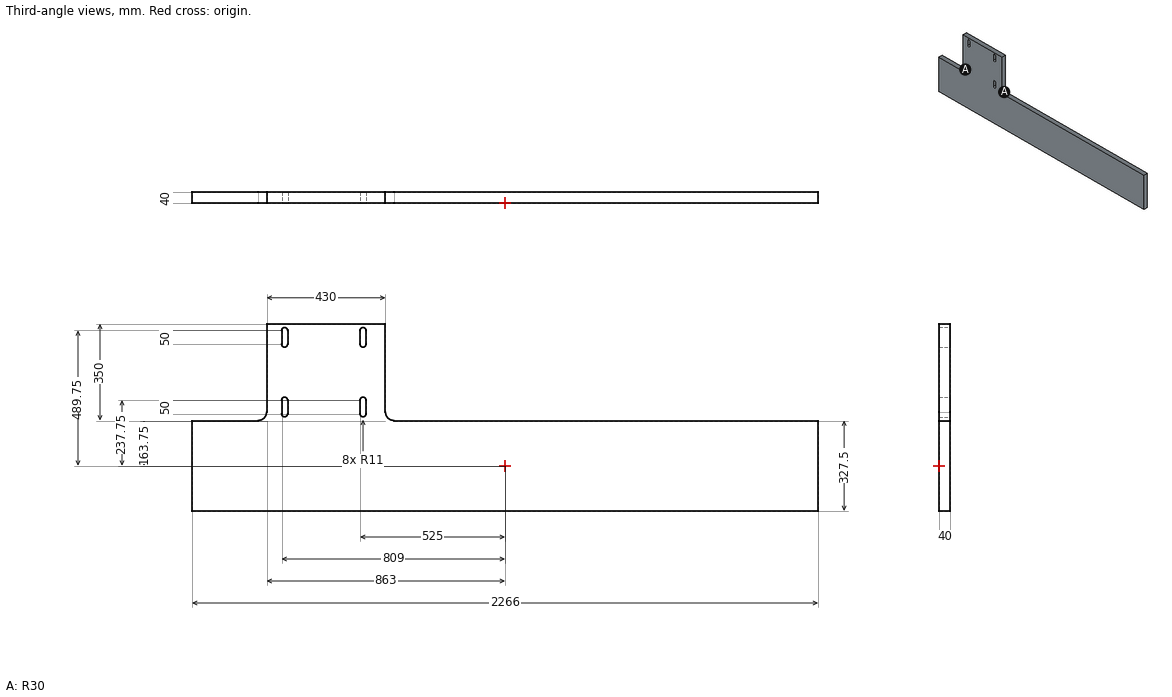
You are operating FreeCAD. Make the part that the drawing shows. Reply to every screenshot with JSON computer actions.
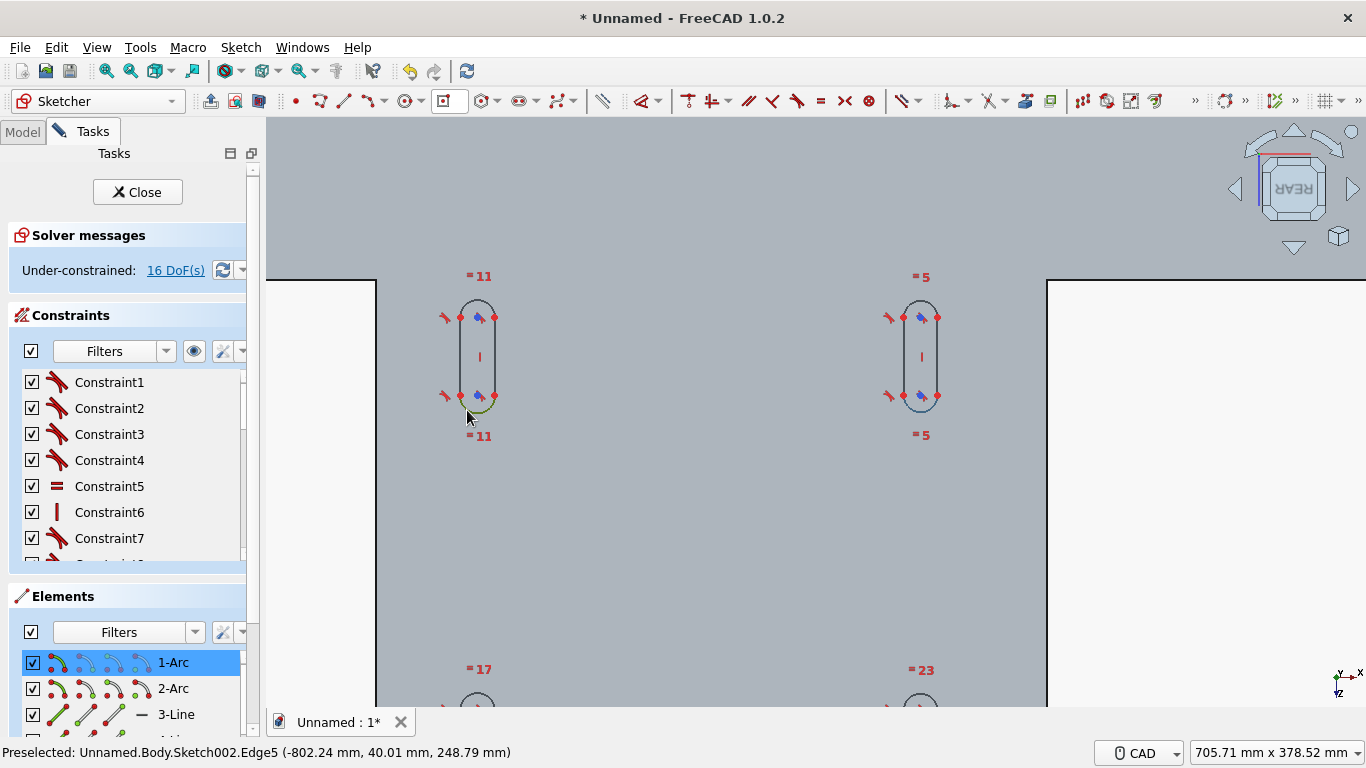
{"action": "scroll", "coordinate": [467, 410], "scroll_direction": "down", "scroll_amount": 4}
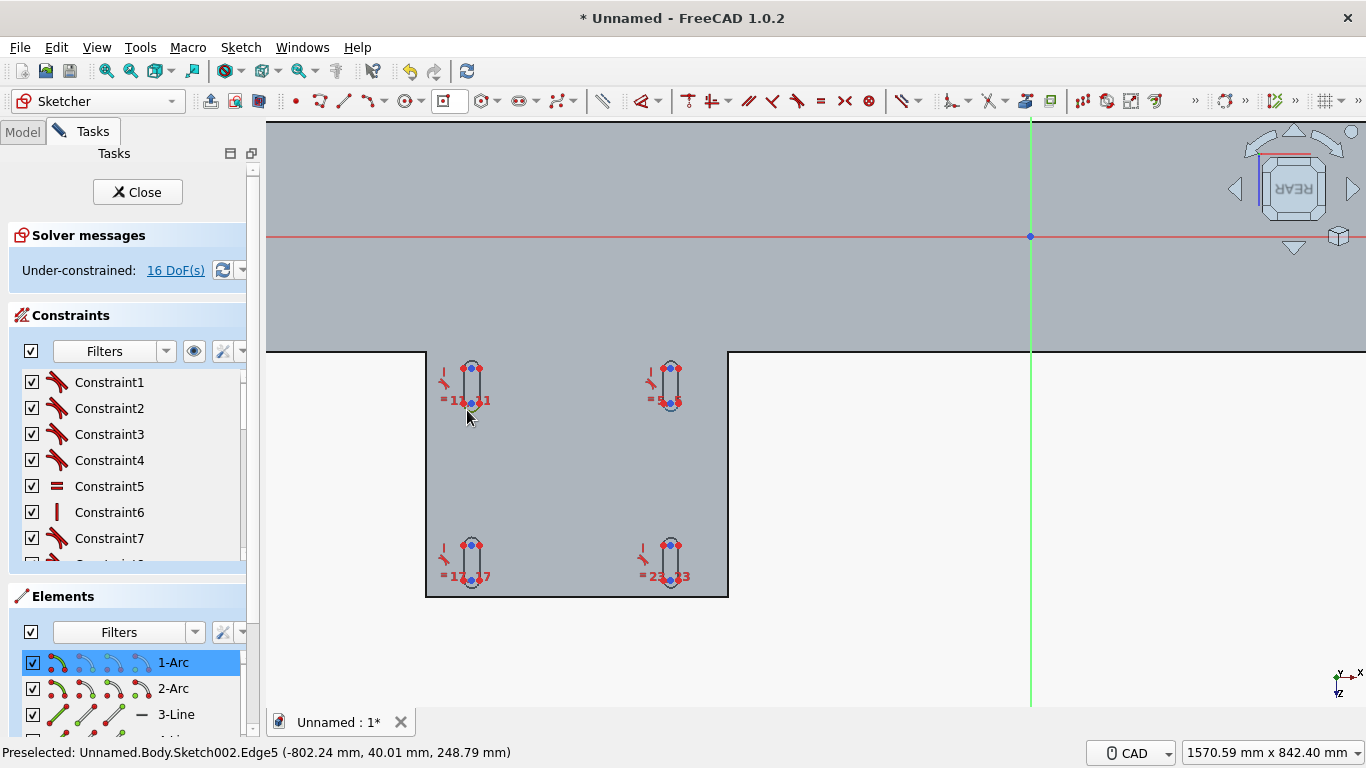
{"action": "scroll", "coordinate": [467, 587], "scroll_direction": "up", "scroll_amount": 4}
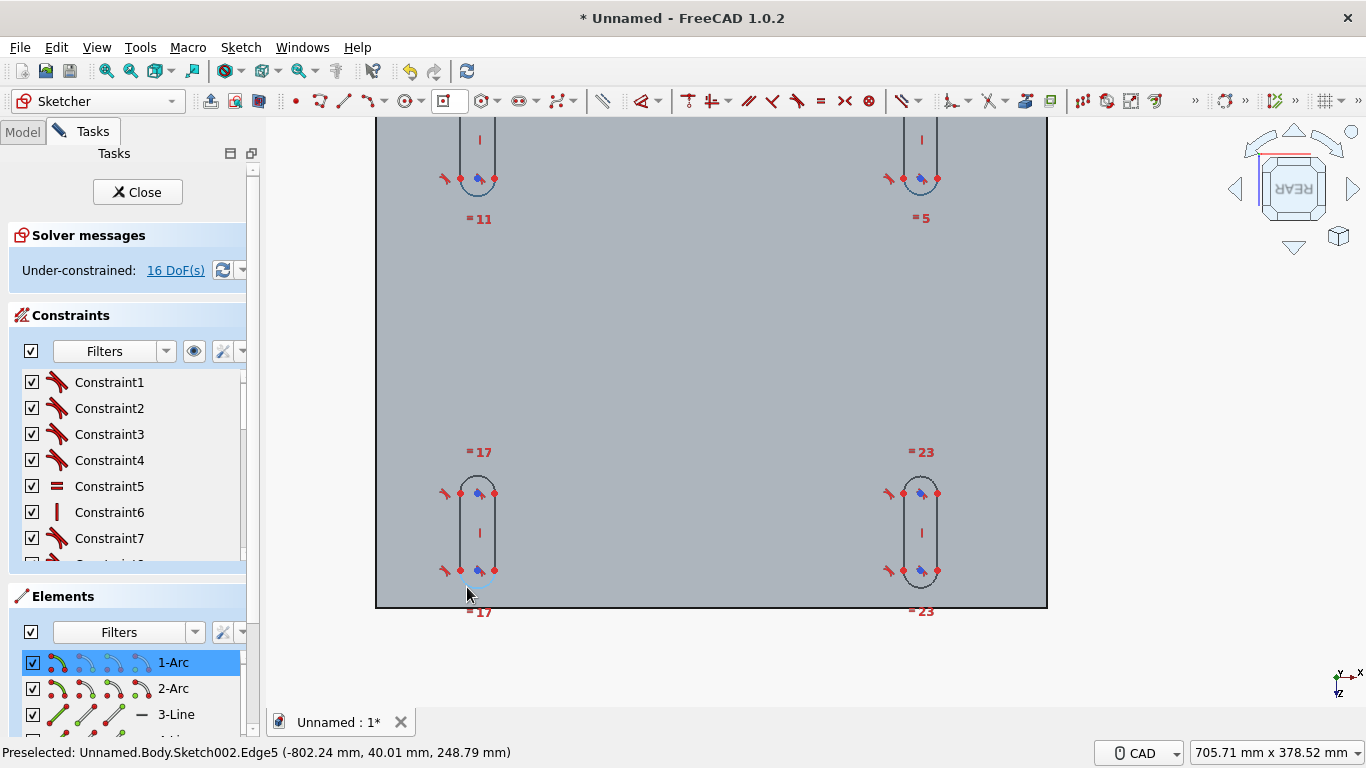
{"action": "left_click", "coordinate": [467, 585]}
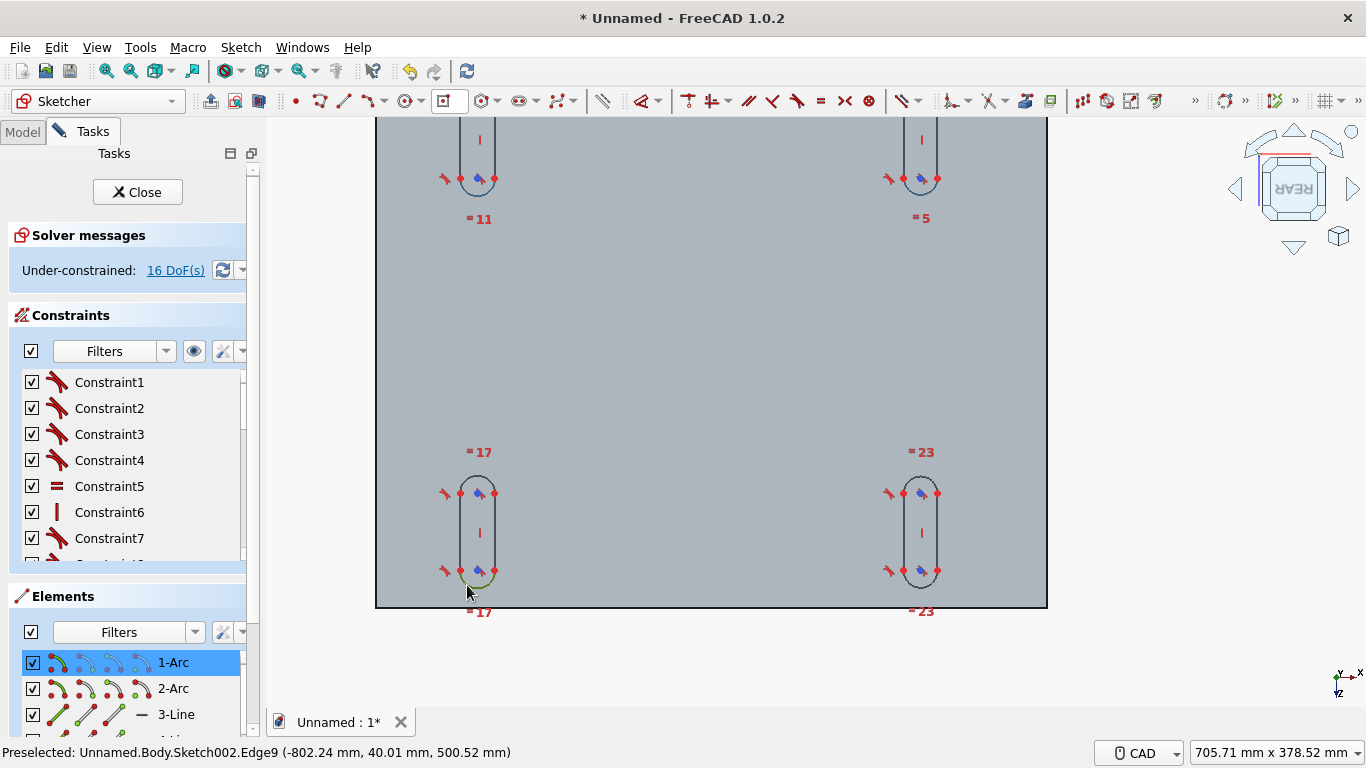
{"action": "left_click", "coordinate": [911, 585]}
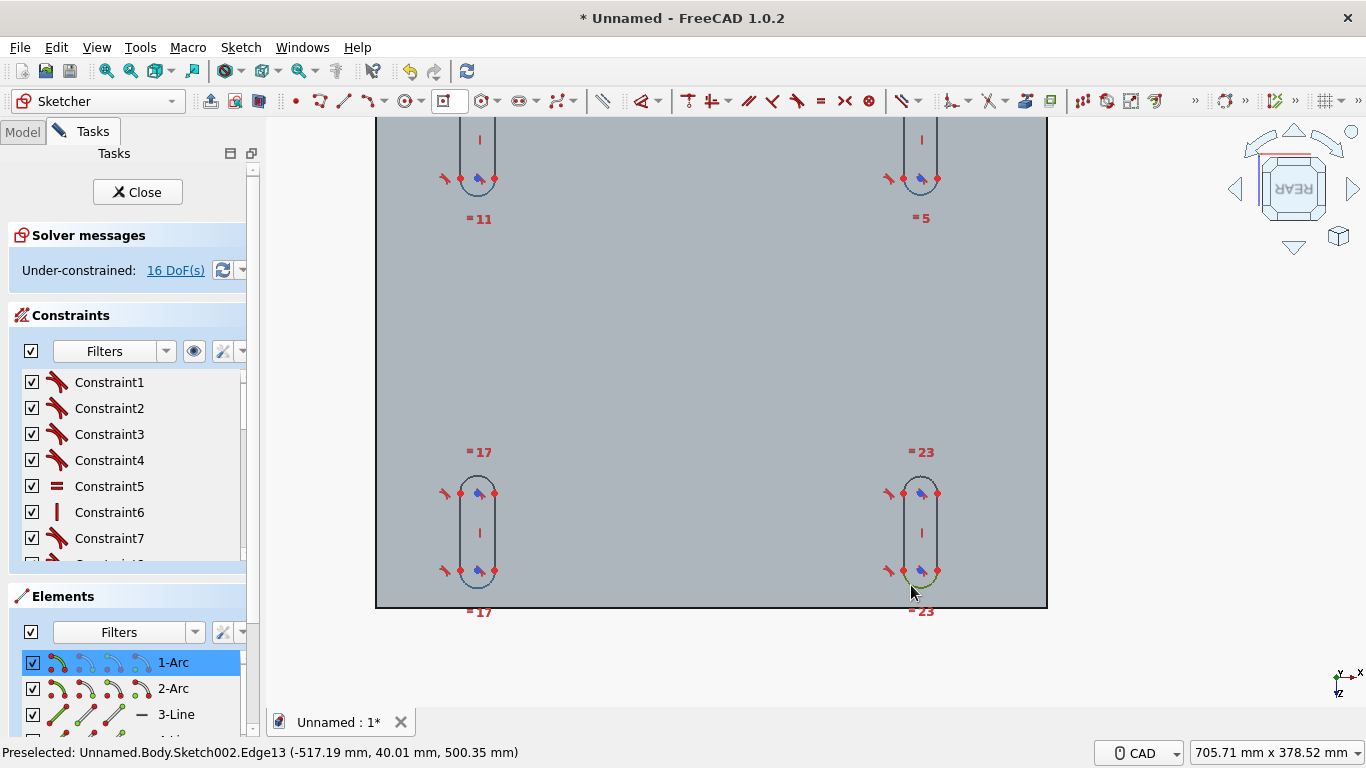
{"action": "left_click", "coordinate": [822, 102]}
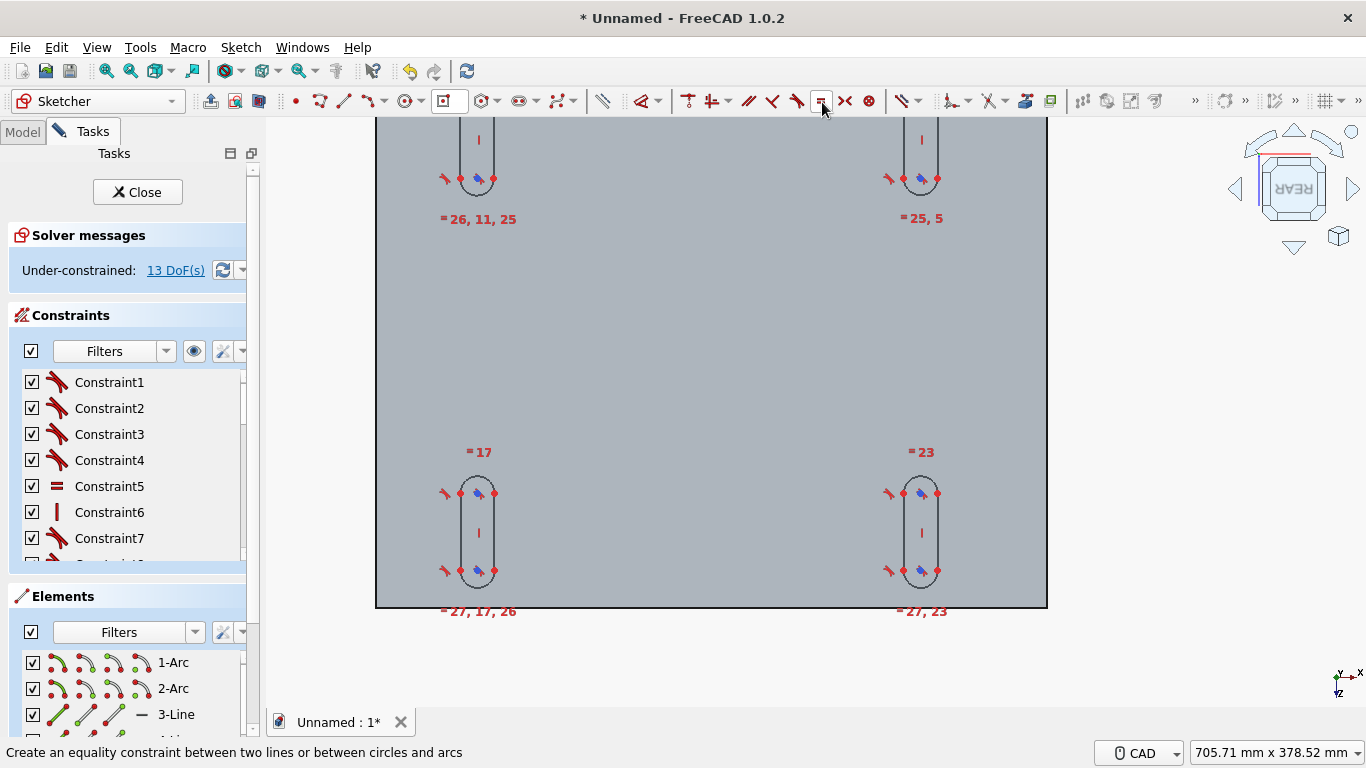
{"action": "left_click", "coordinate": [642, 102]}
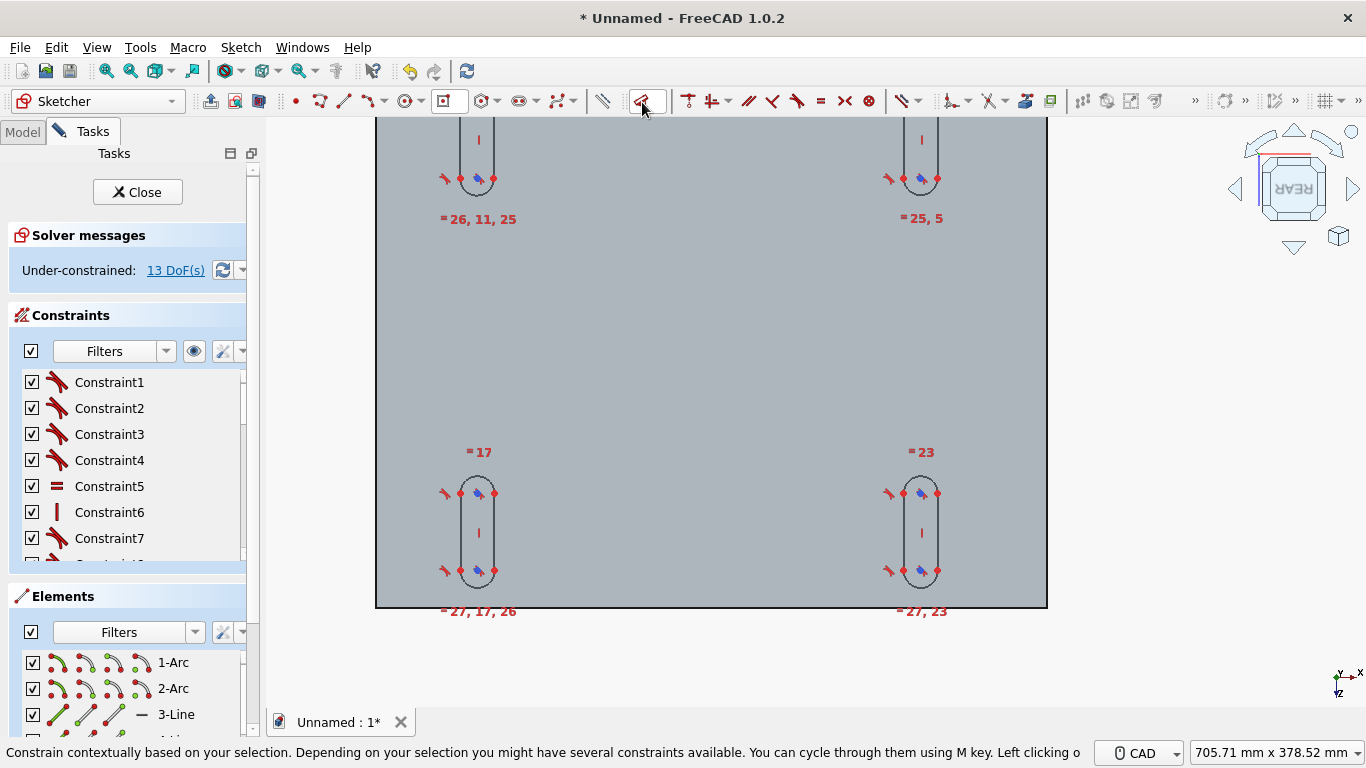
{"action": "scroll", "coordinate": [911, 192], "scroll_direction": "up", "scroll_amount": 5}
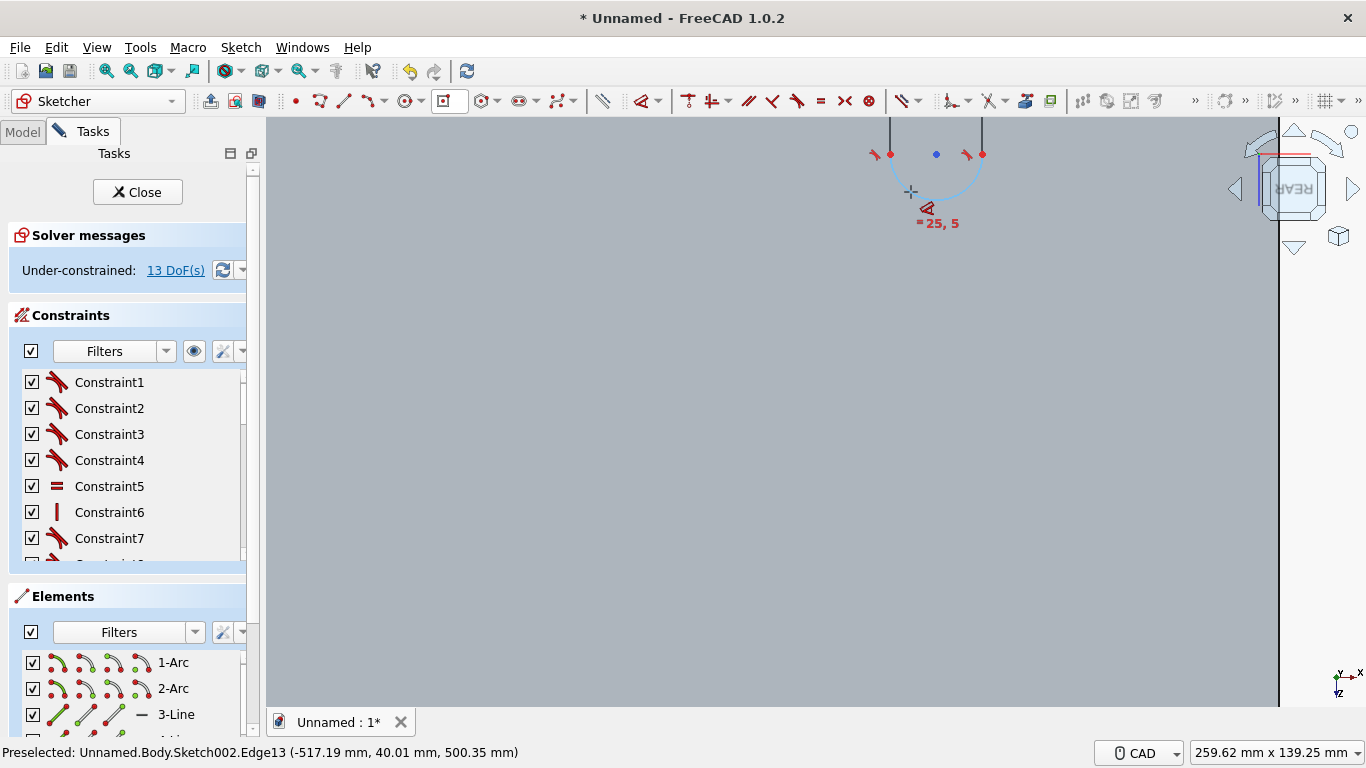
{"action": "left_click", "coordinate": [909, 191]}
{"action": "left_click", "coordinate": [890, 217]}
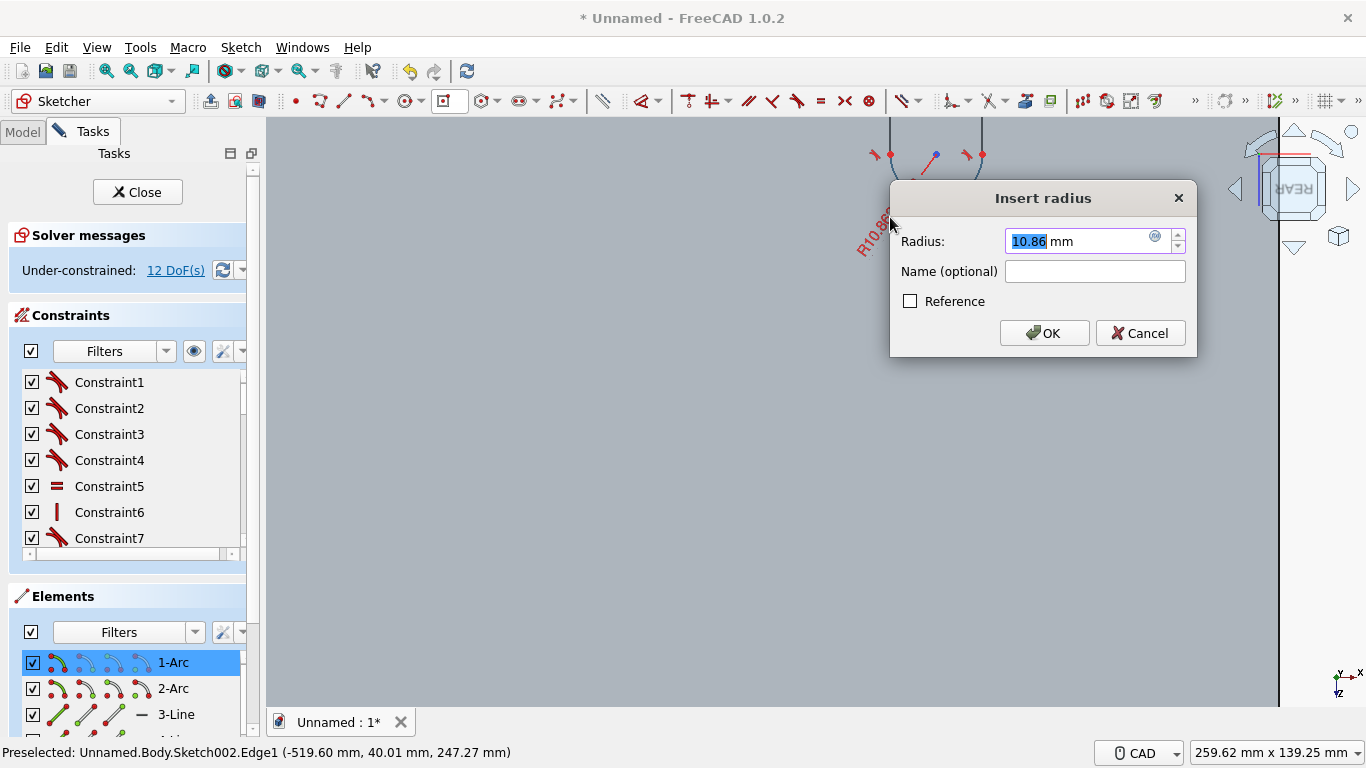
{"action": "type", "text": "11"}
{"action": "key", "text": "Return"}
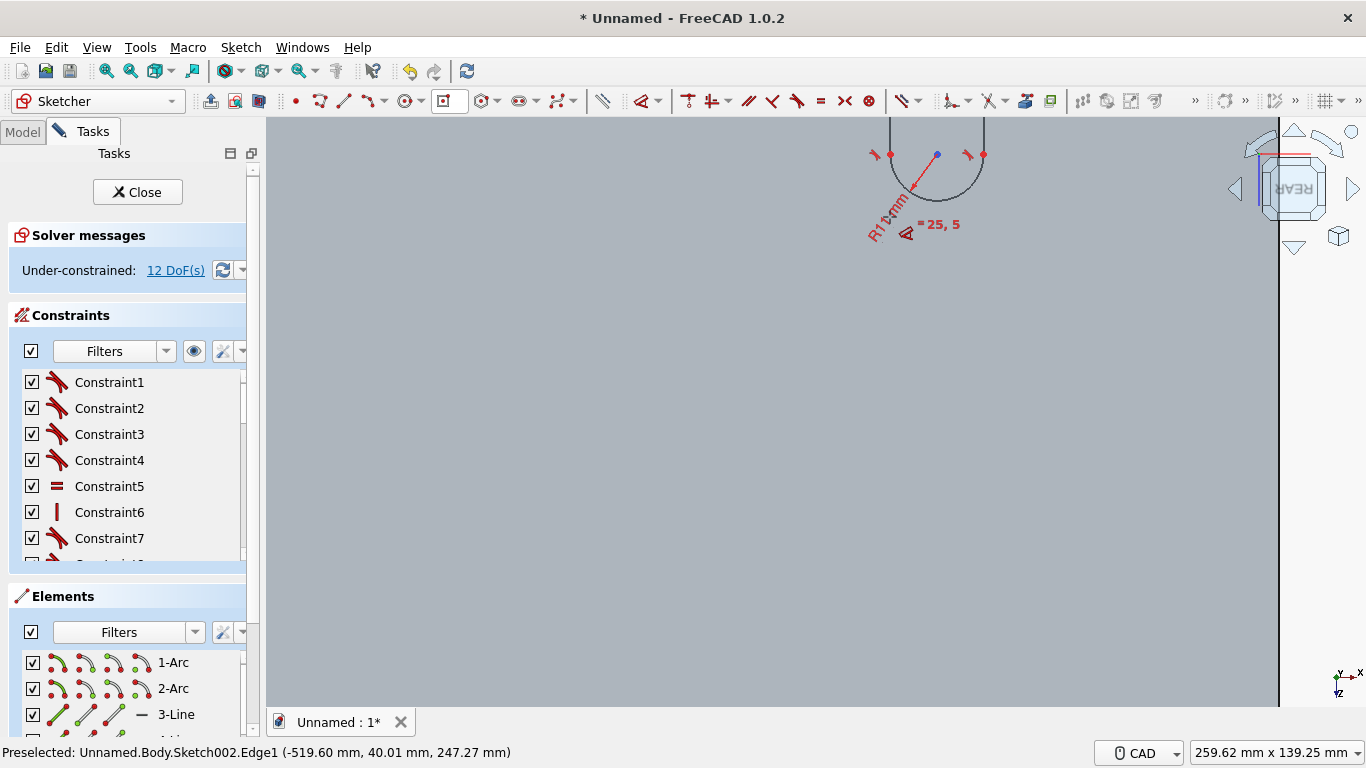
{"action": "scroll", "coordinate": [618, 453], "scroll_direction": "down", "scroll_amount": 9}